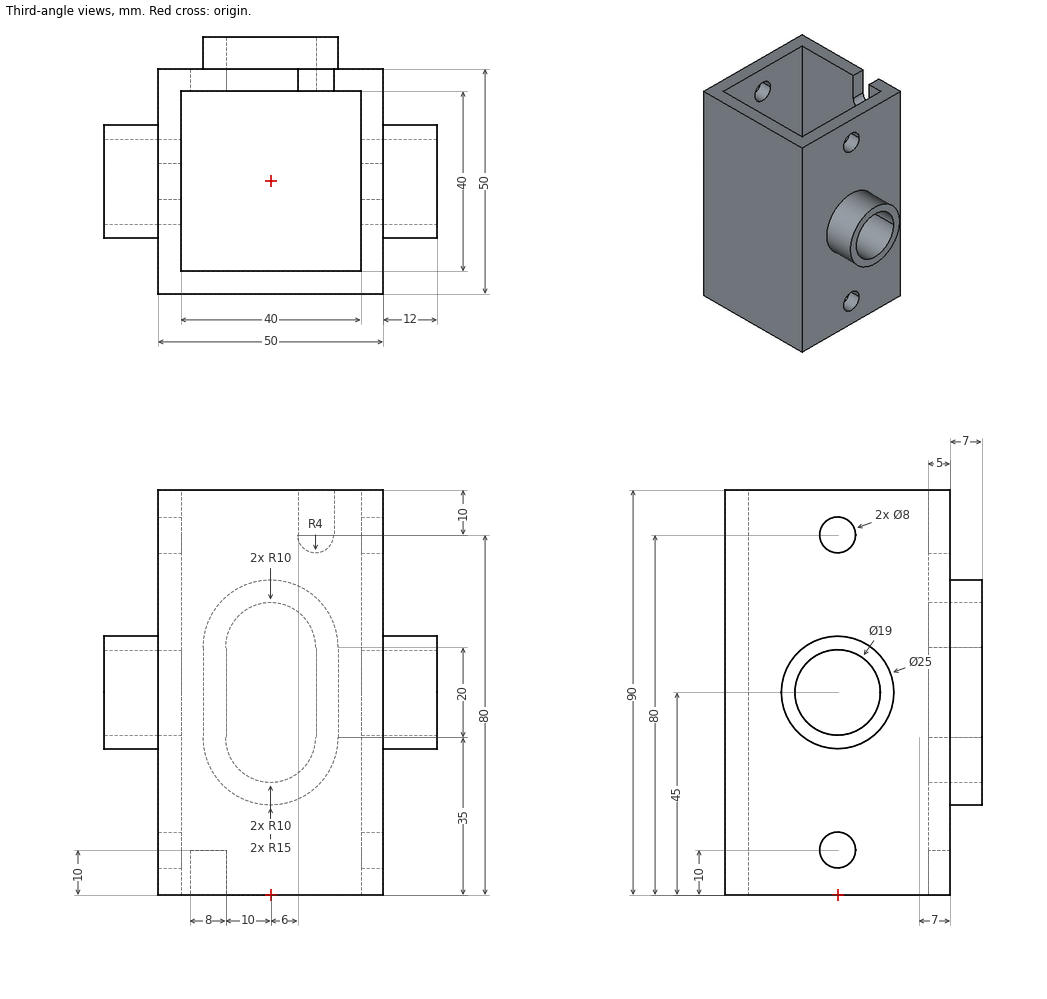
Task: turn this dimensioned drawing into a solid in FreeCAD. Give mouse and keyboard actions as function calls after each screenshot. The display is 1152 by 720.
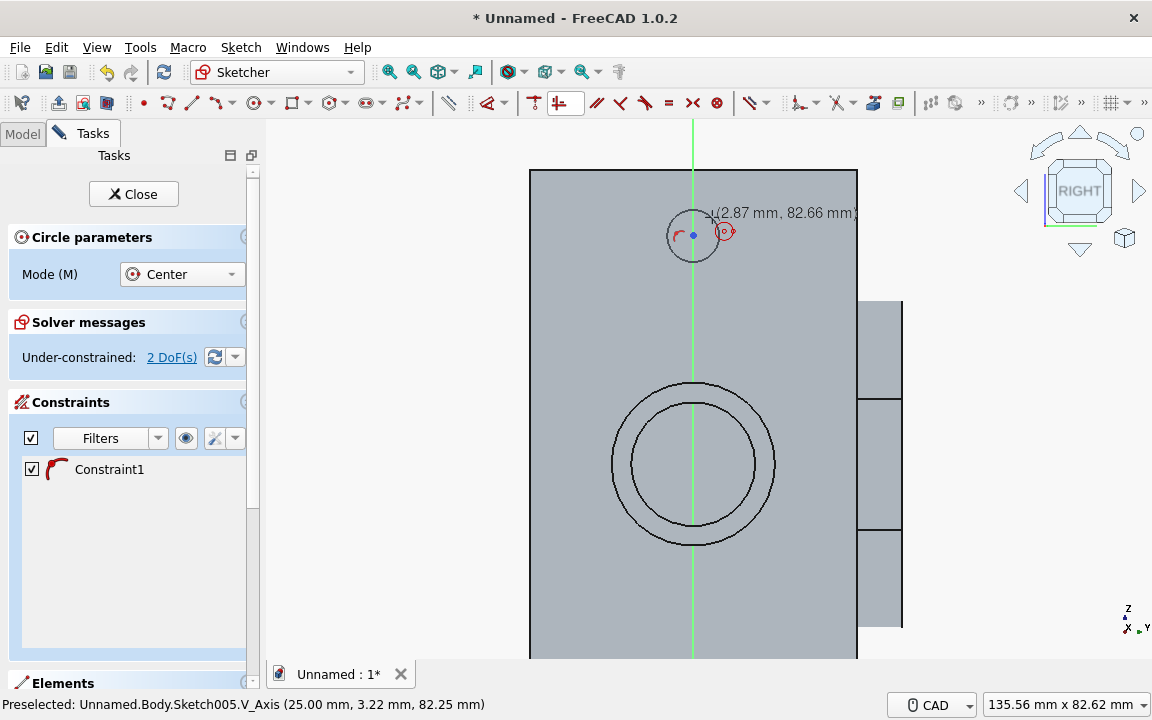
scroll(533, 196, down, 2)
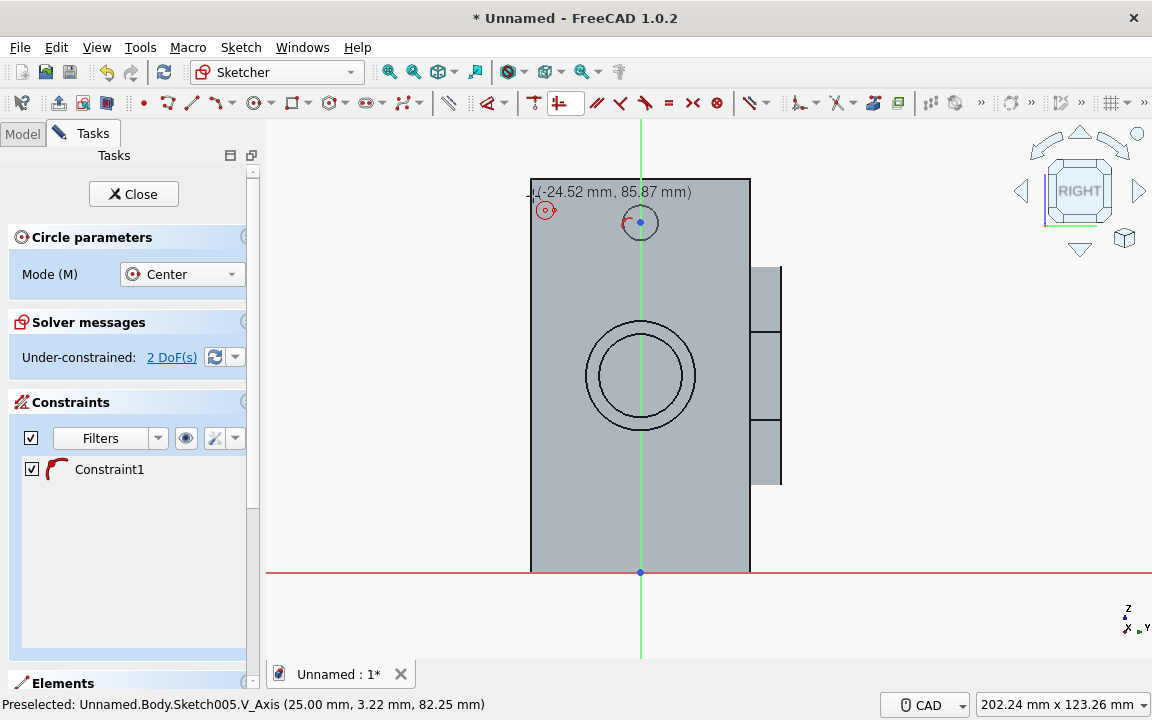
scroll(641, 529, up, 2)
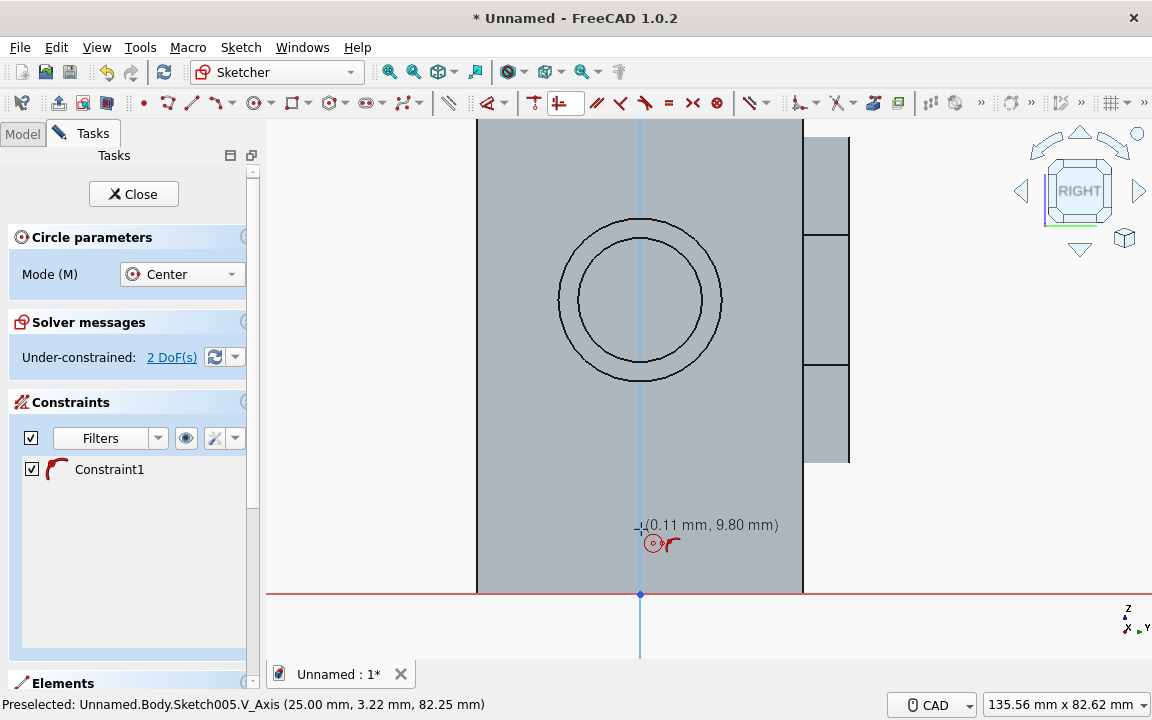
click(640, 529)
click(659, 510)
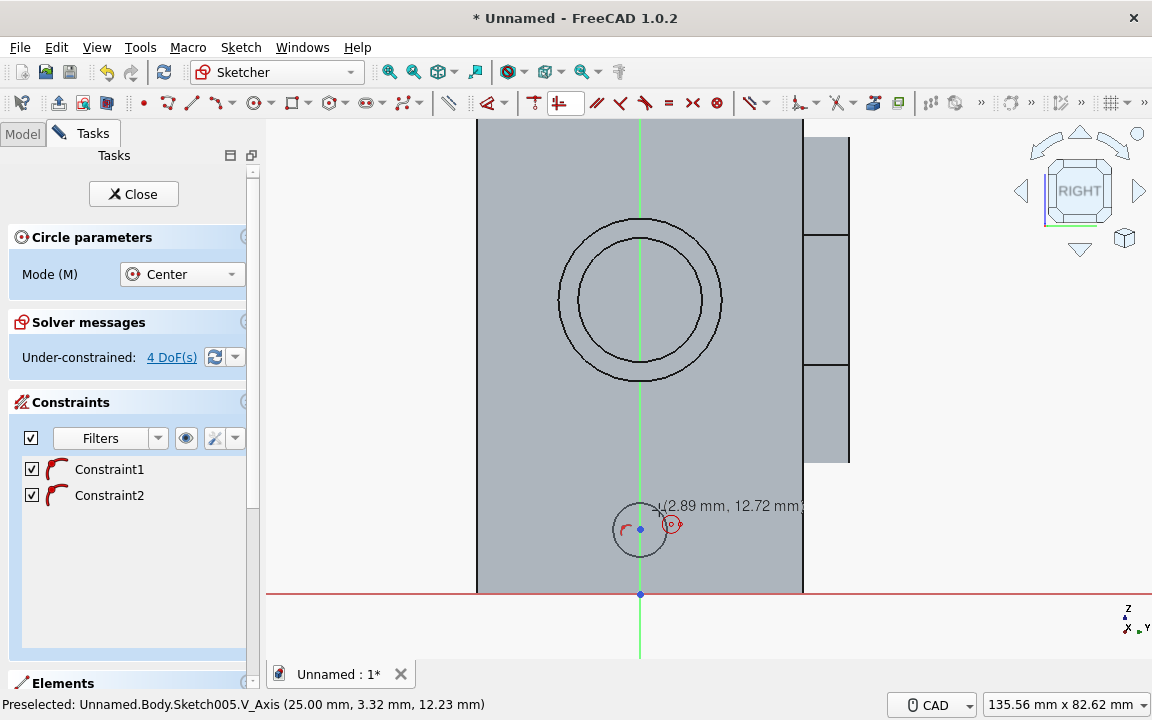
click(640, 300)
click(684, 256)
key(Escape)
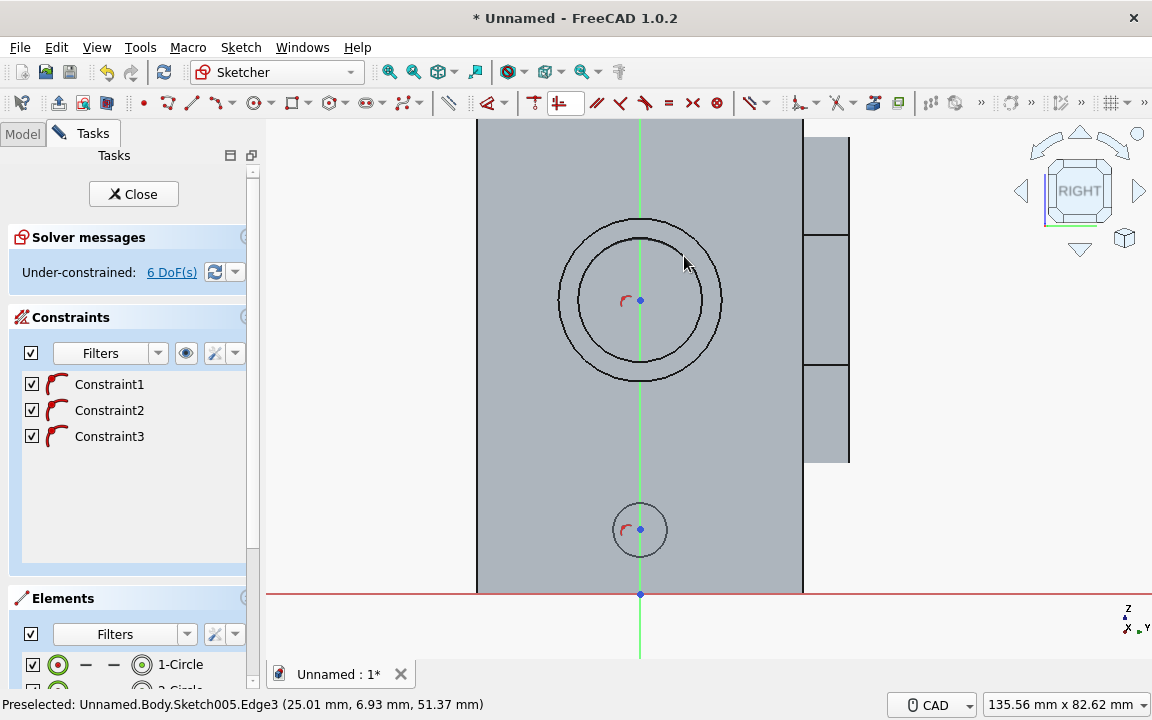
scroll(641, 530, down, 2)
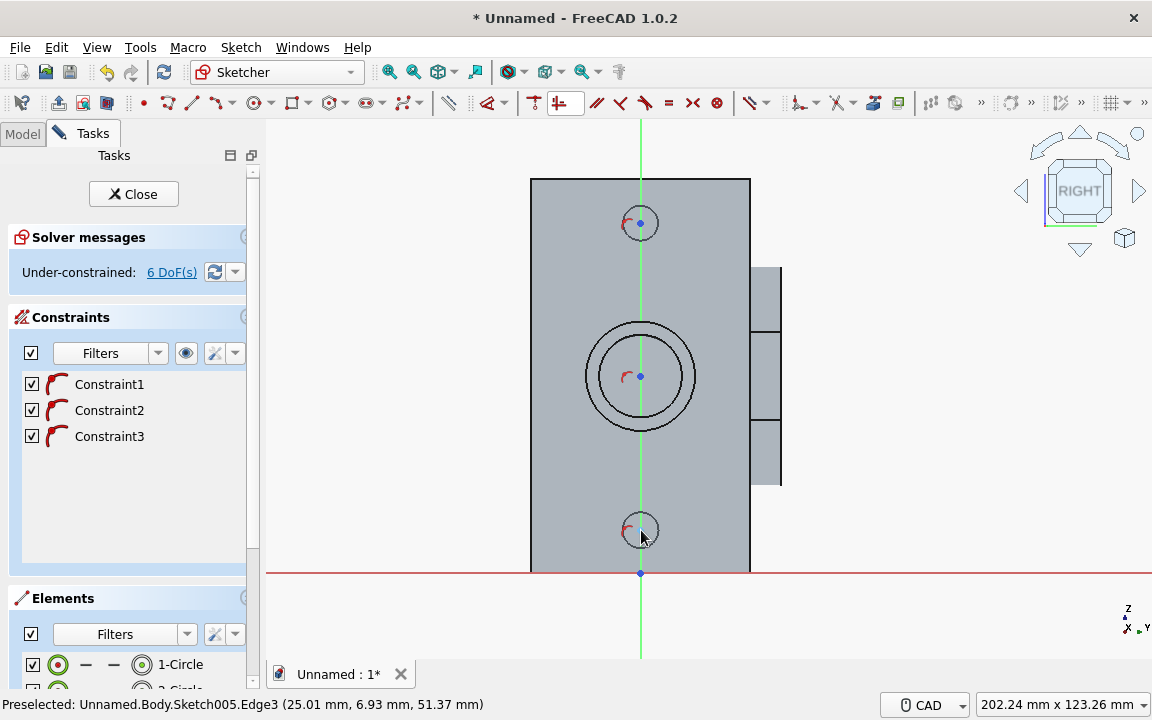
click(653, 211)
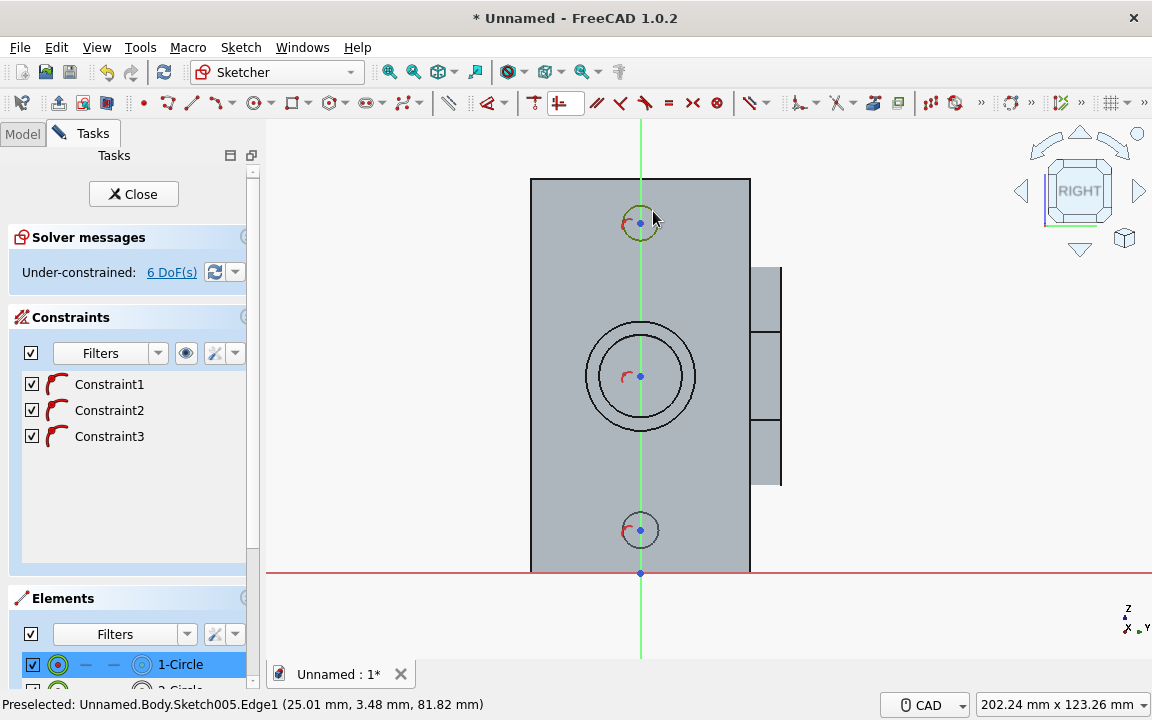
click(653, 518)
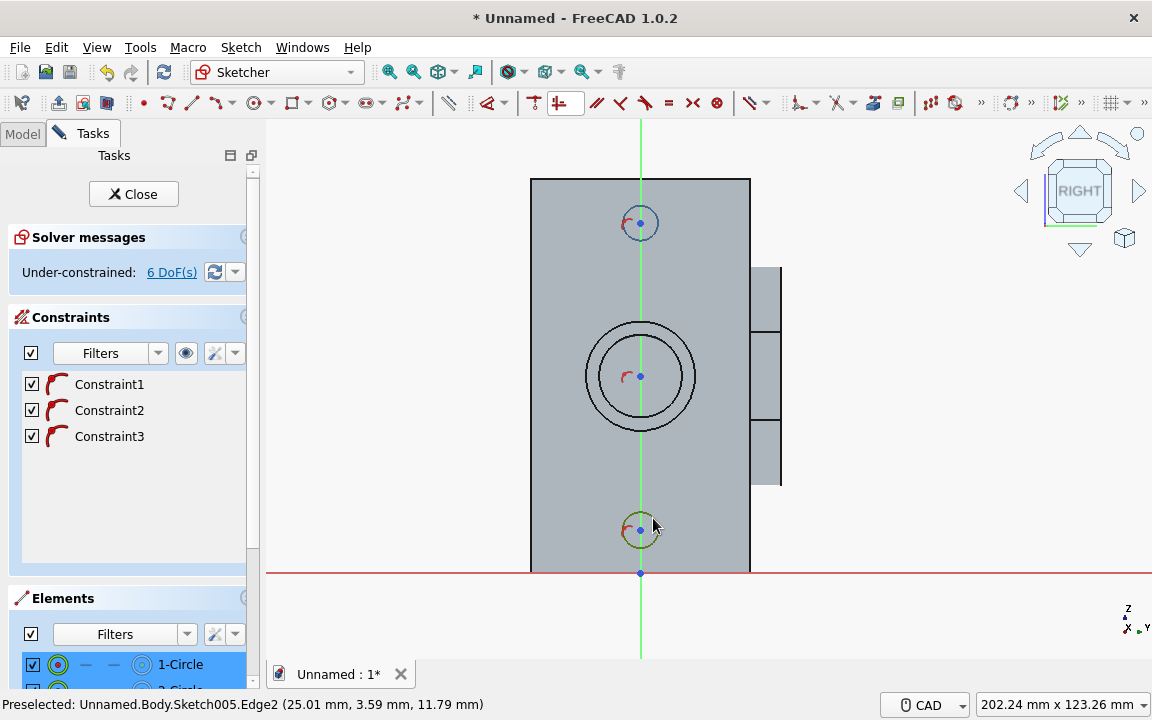
key(e)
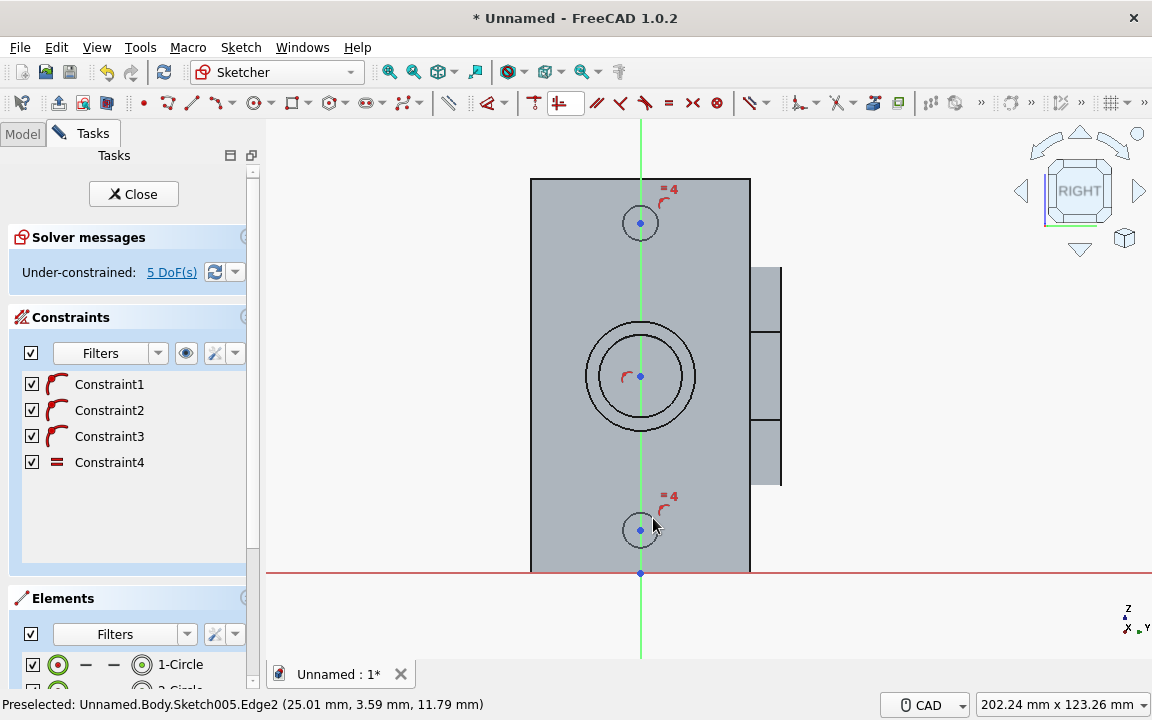
click(488, 104)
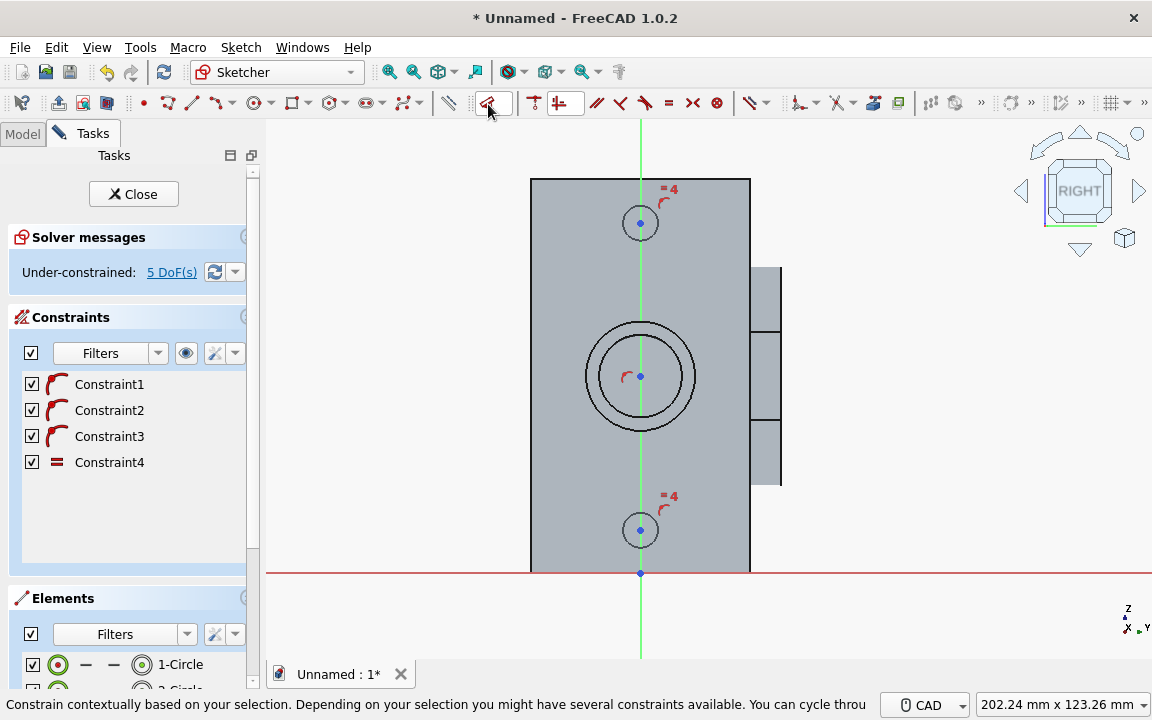
click(653, 211)
click(676, 189)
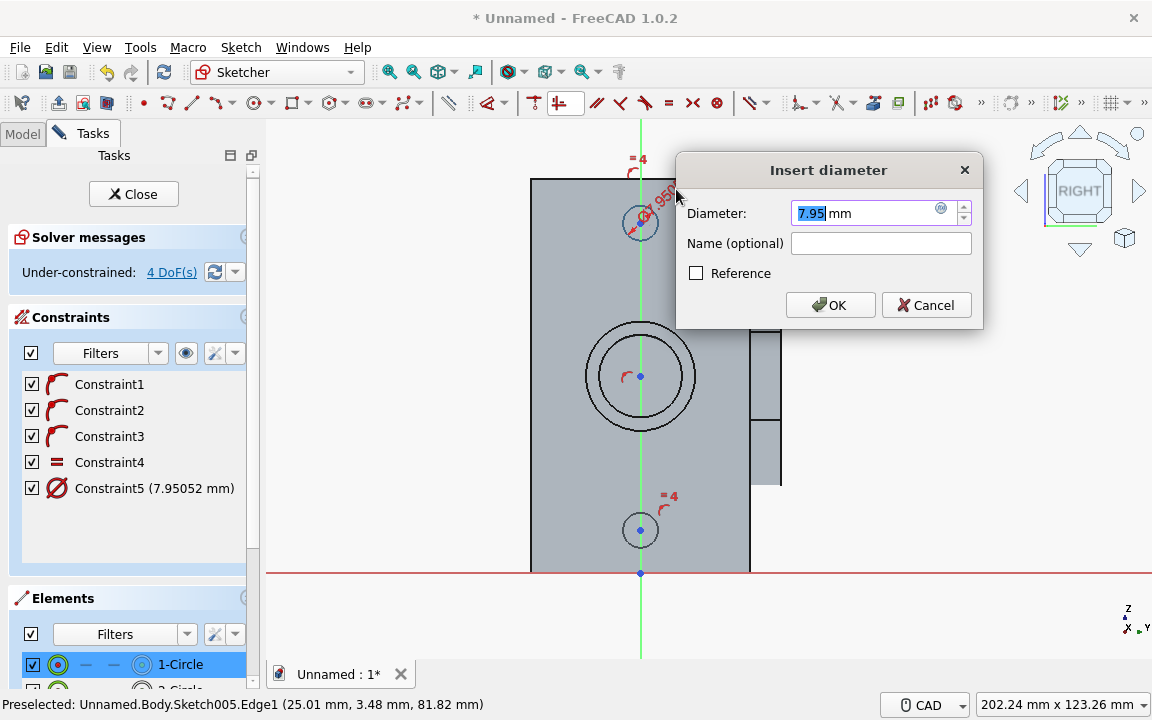
text(8)
key(Return)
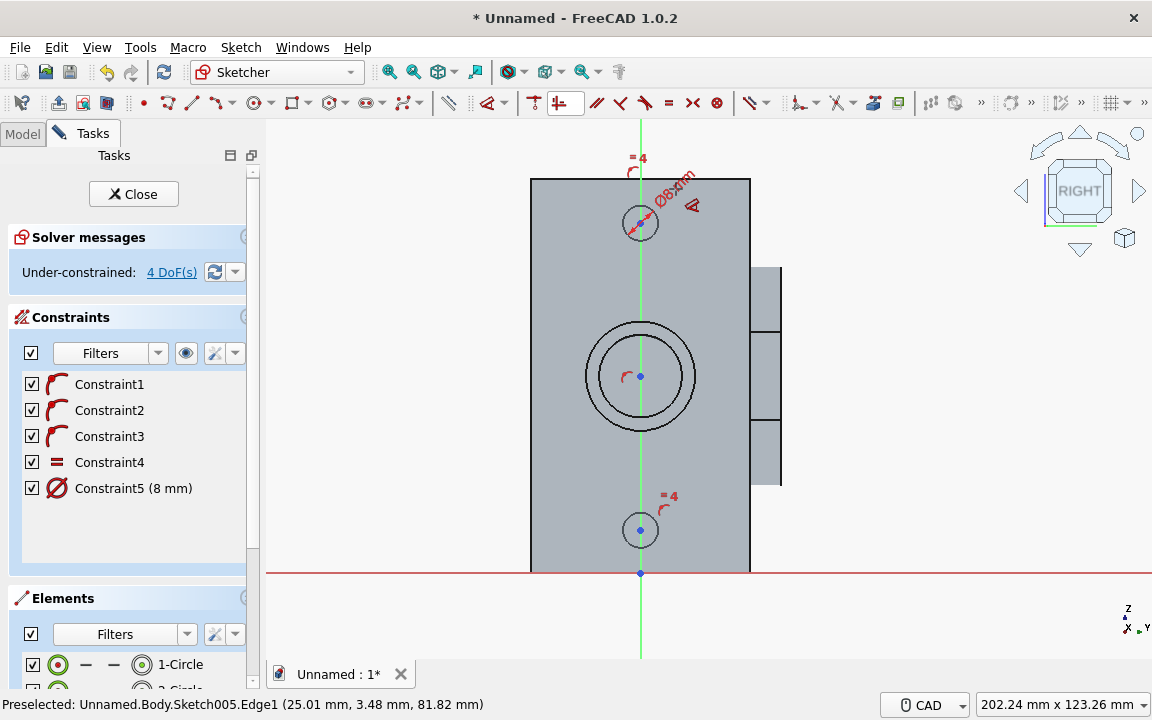
click(670, 347)
click(693, 324)